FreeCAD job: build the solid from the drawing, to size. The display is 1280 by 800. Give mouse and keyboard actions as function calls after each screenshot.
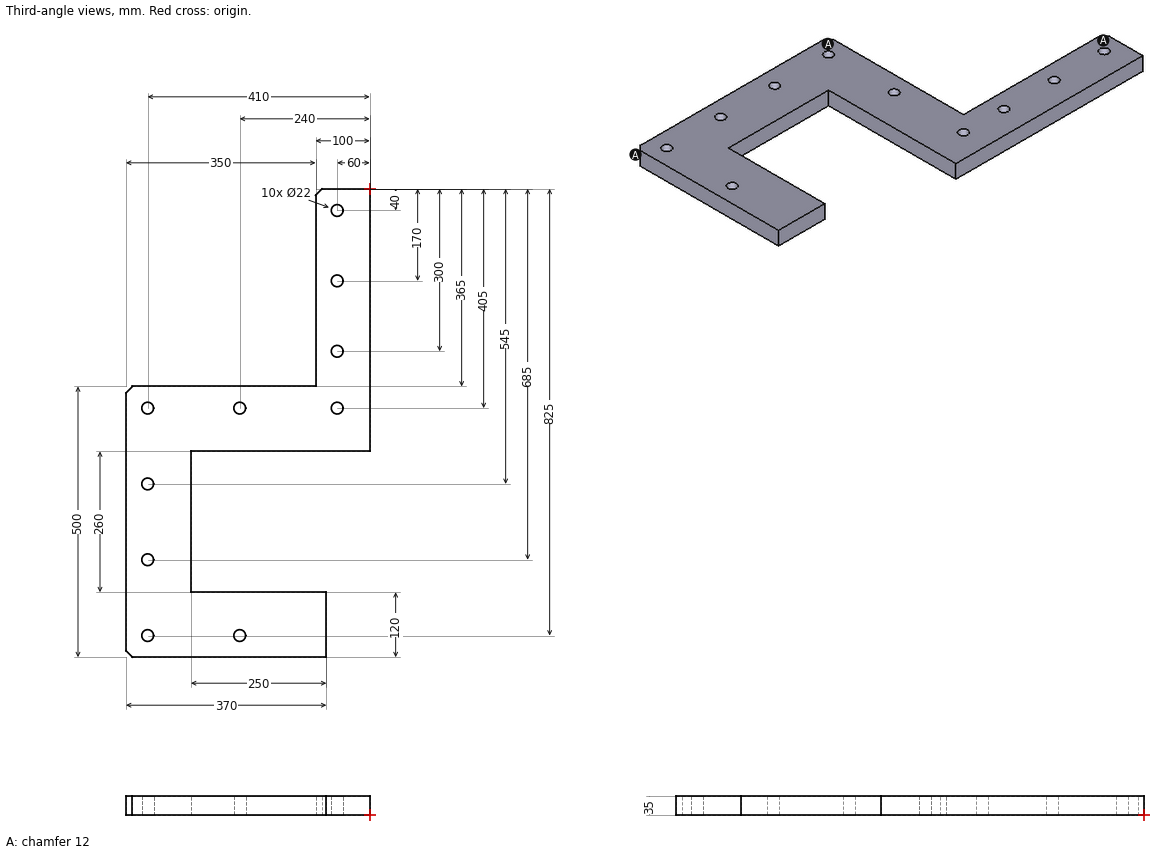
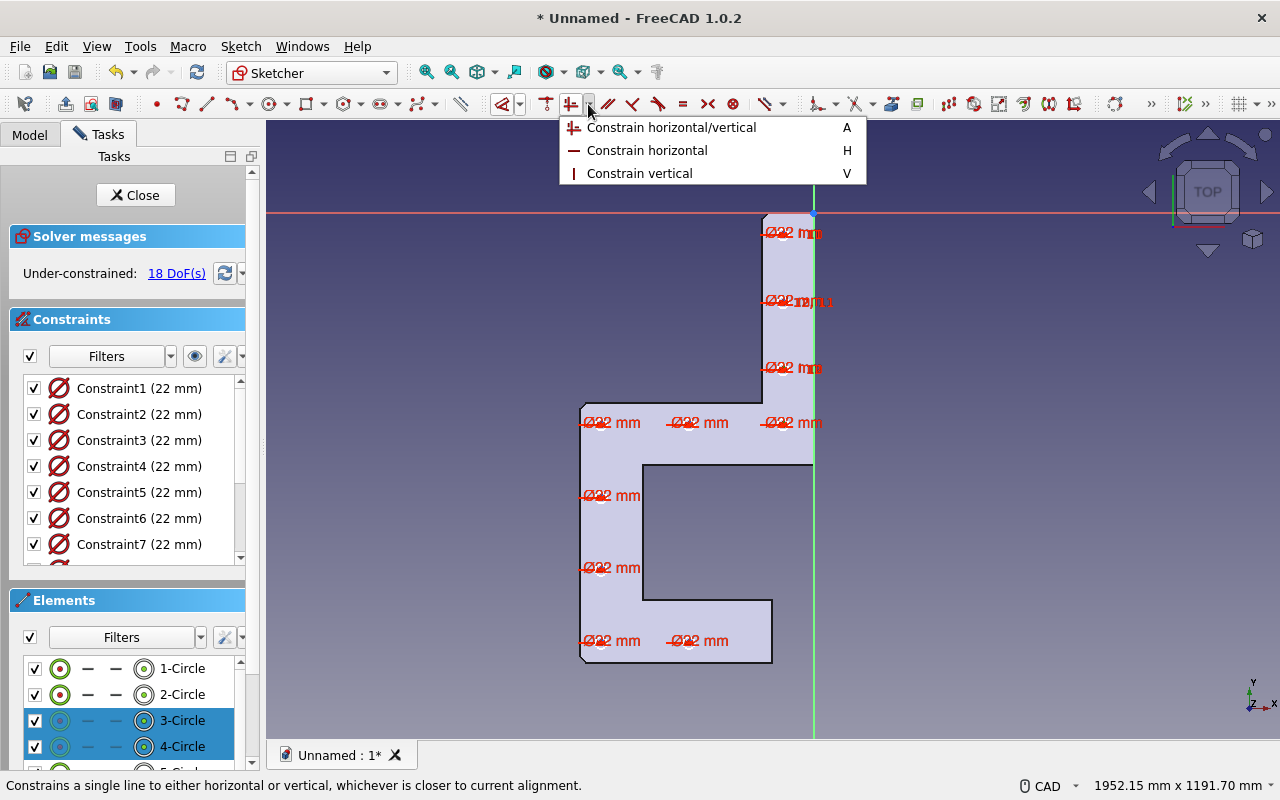
click(713, 174)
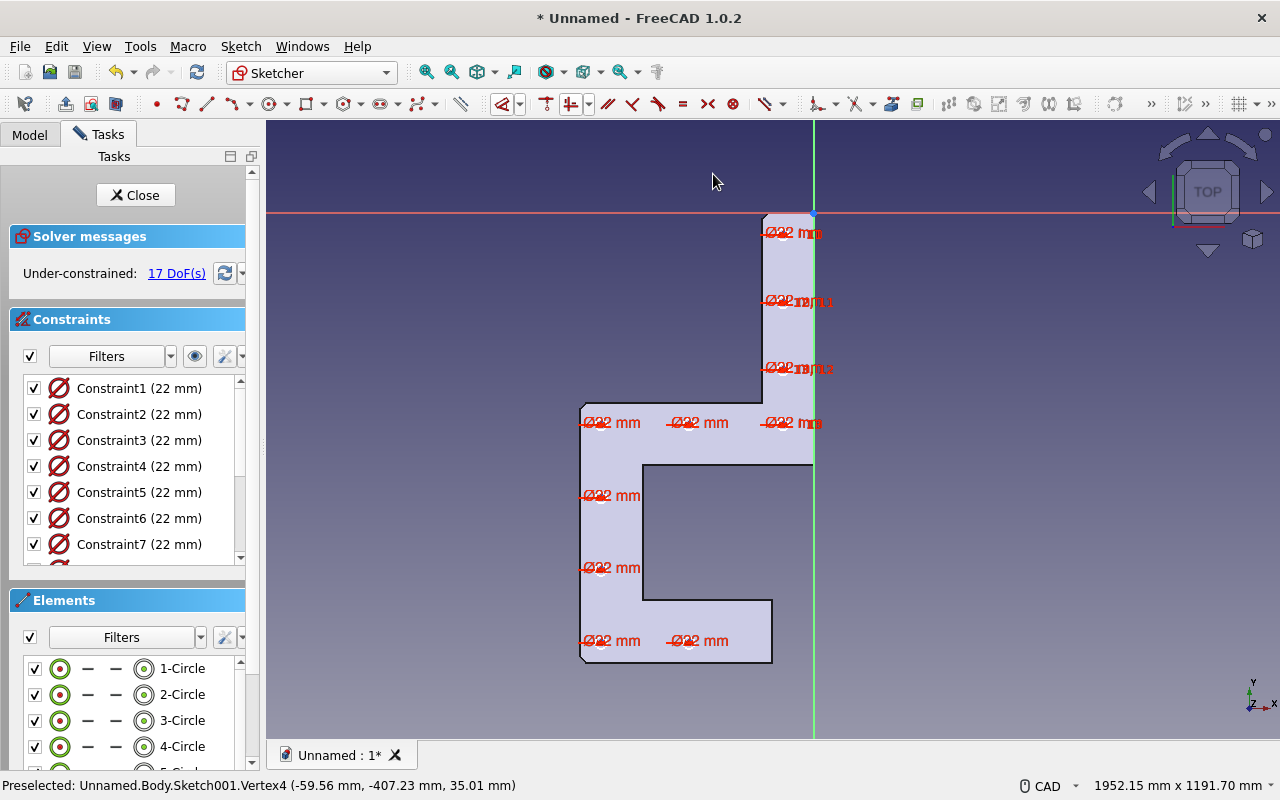
click(783, 425)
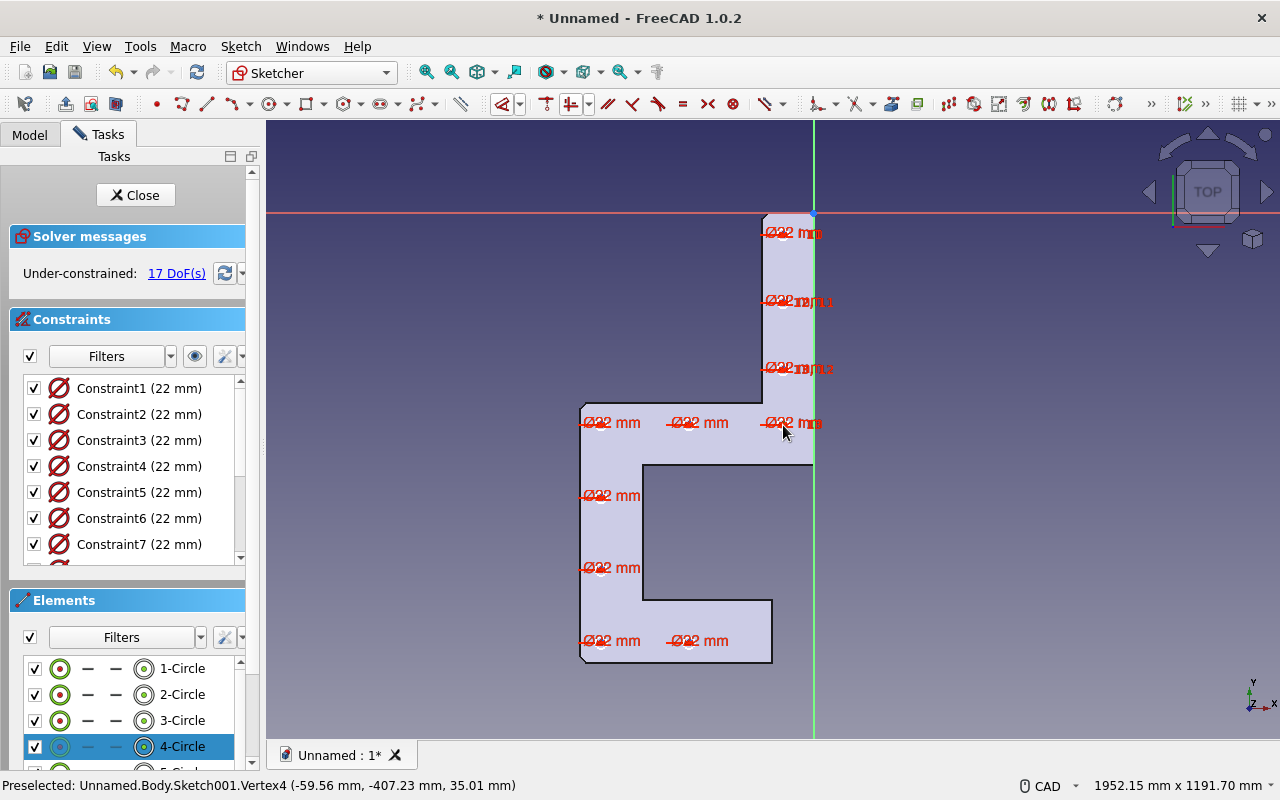
click(689, 425)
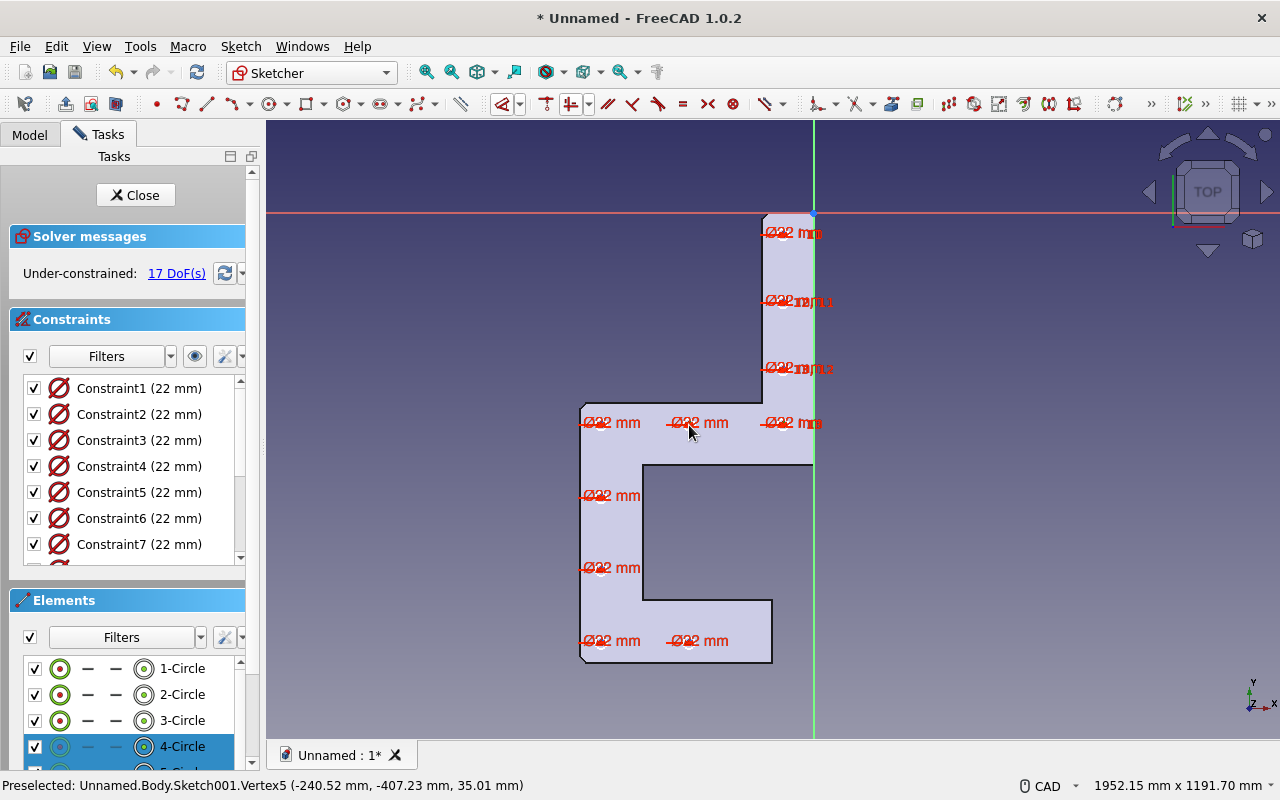
click(588, 104)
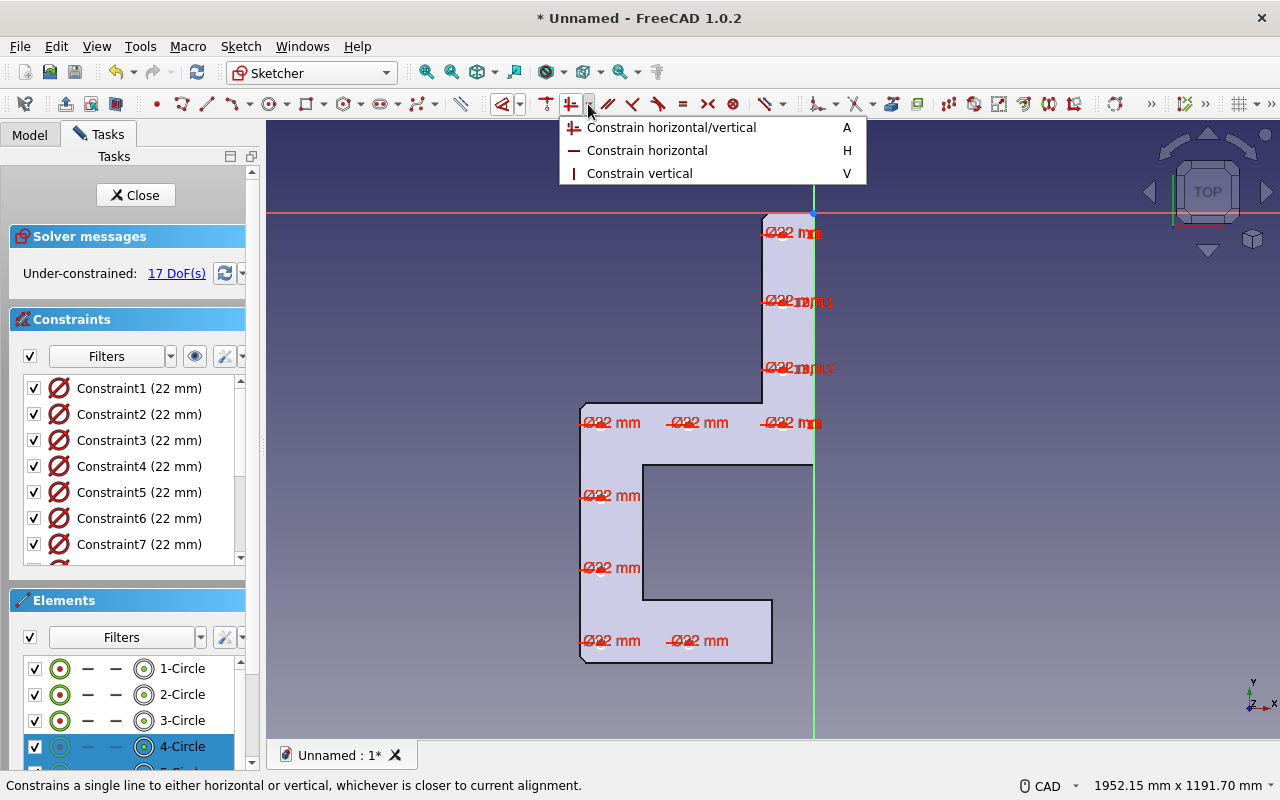
click(713, 150)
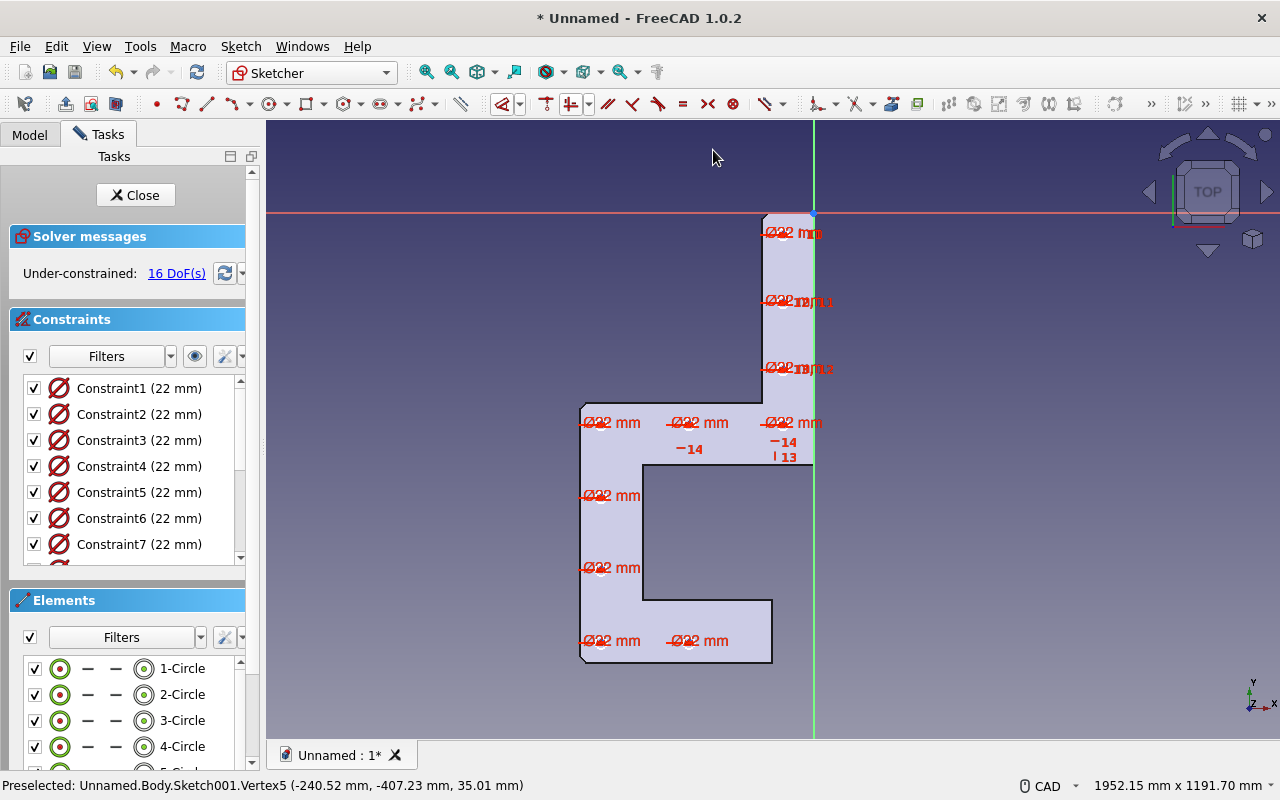
click(689, 425)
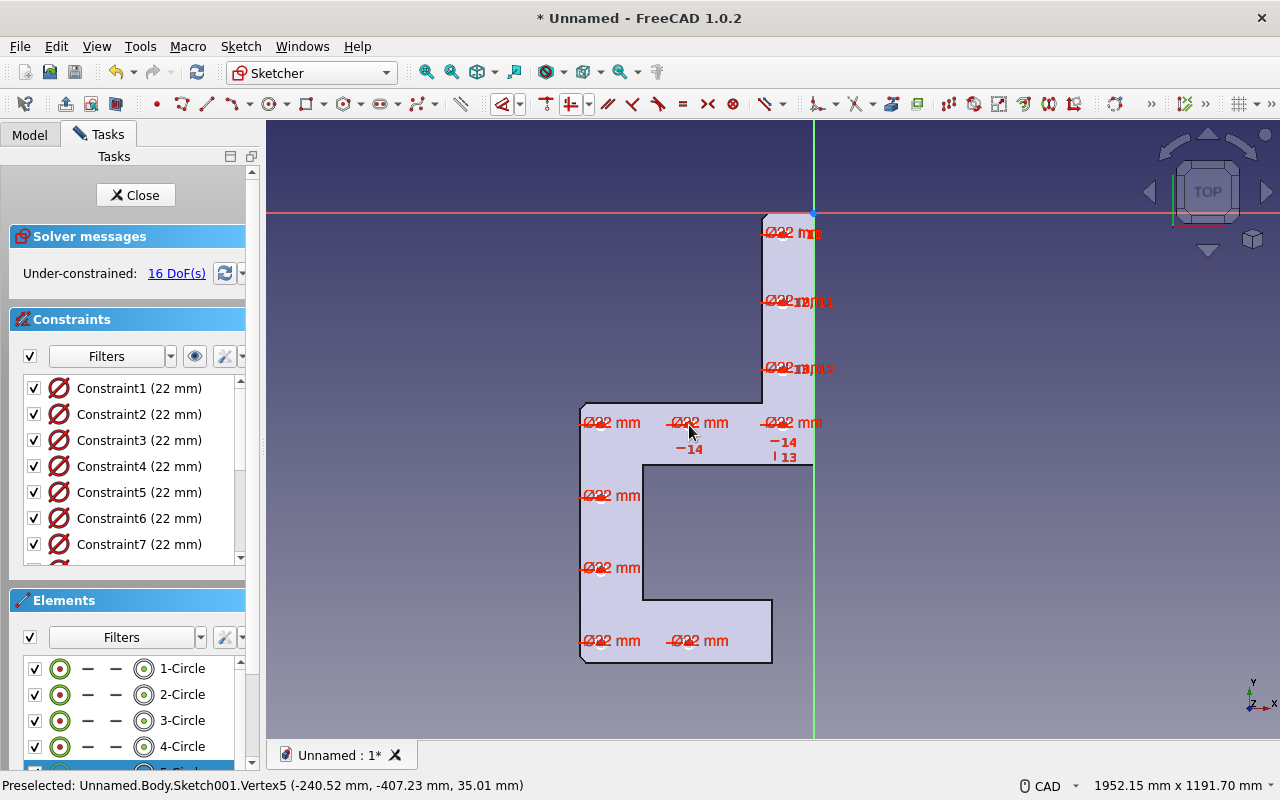
click(601, 425)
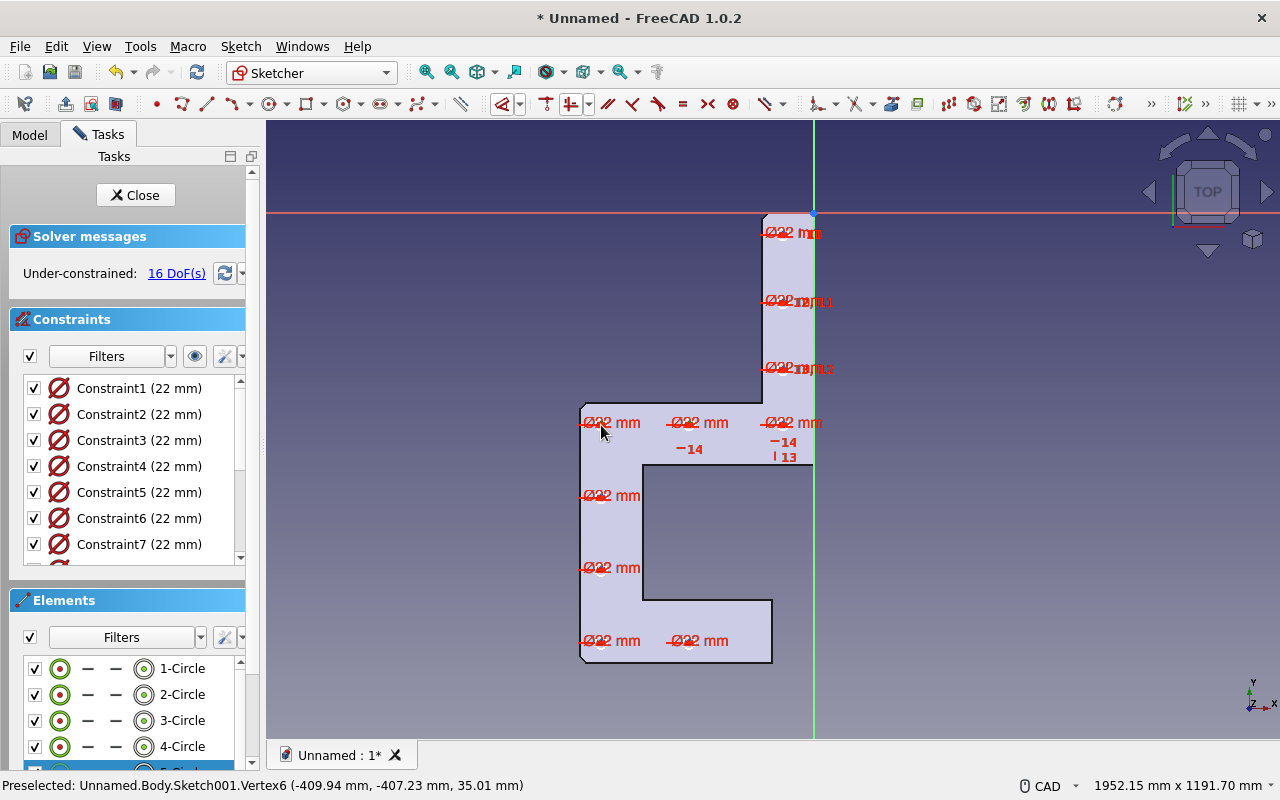
key(h)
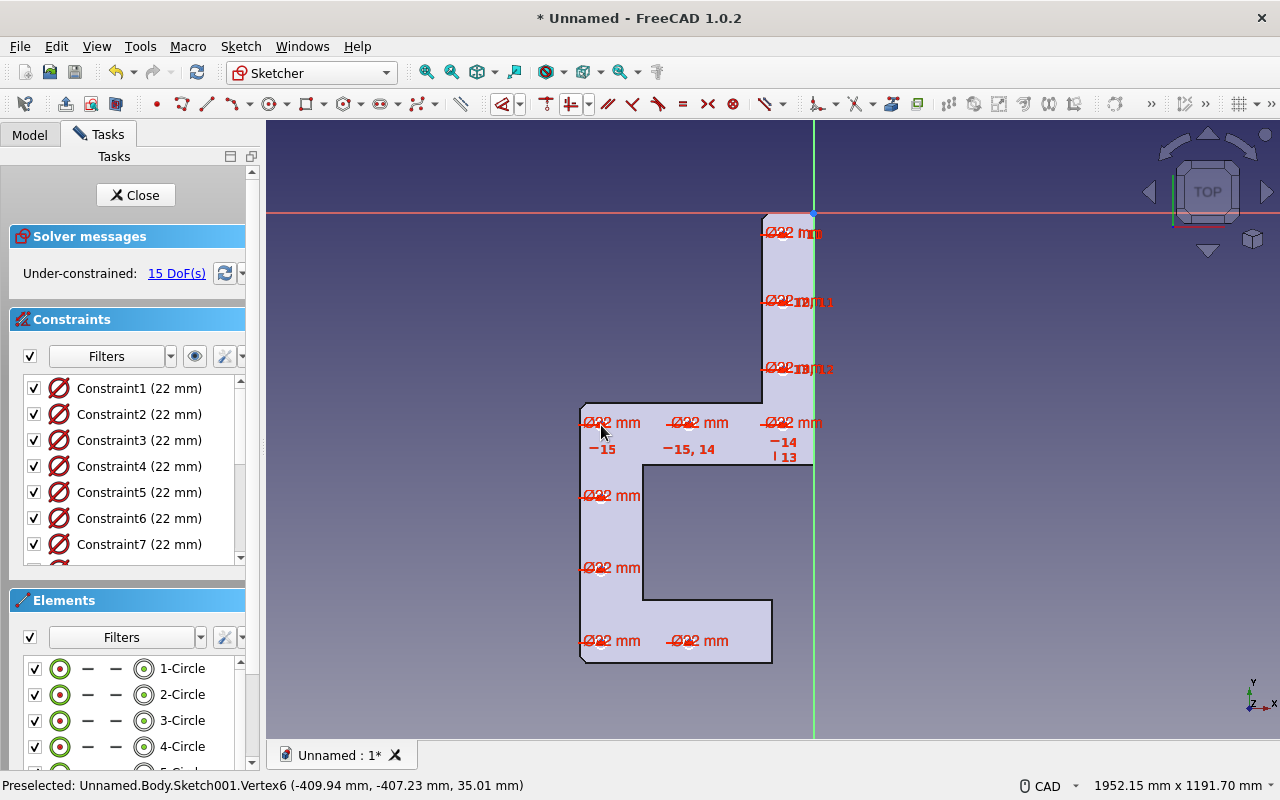
click(601, 425)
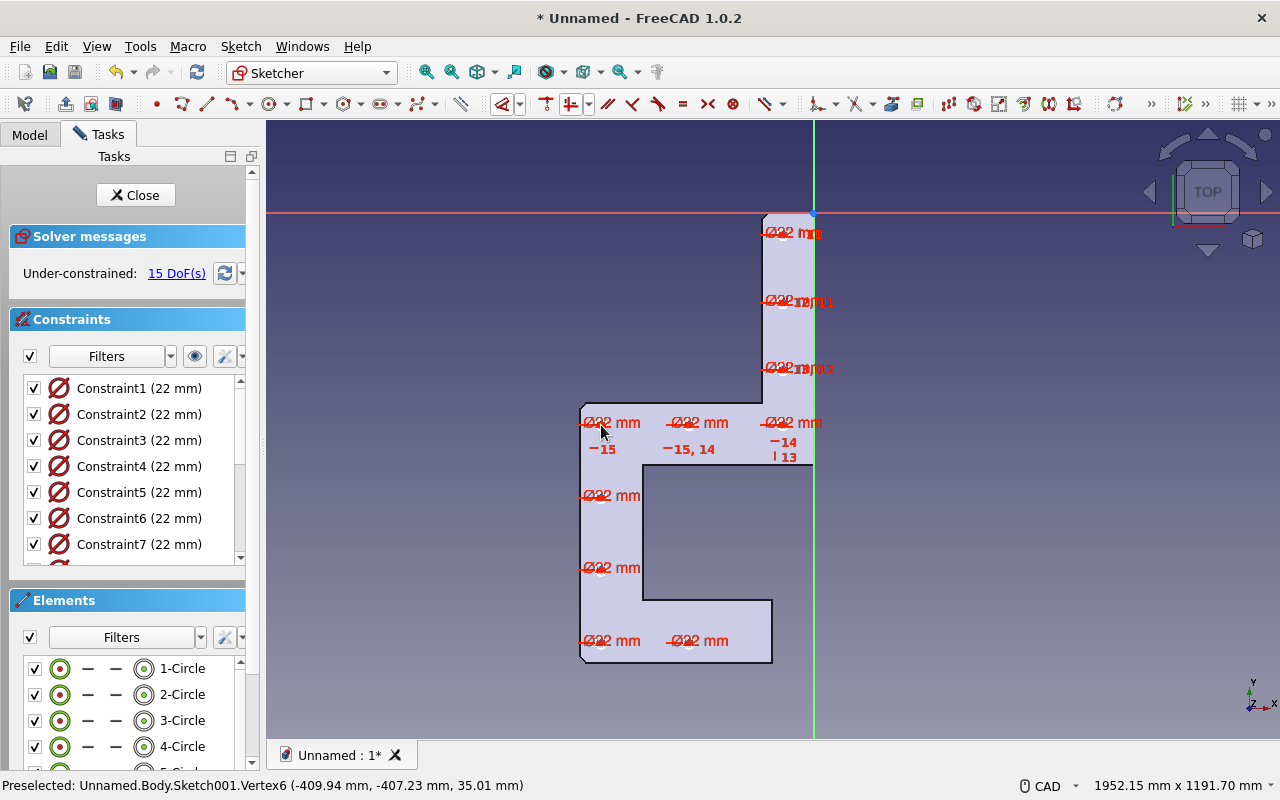
click(601, 498)